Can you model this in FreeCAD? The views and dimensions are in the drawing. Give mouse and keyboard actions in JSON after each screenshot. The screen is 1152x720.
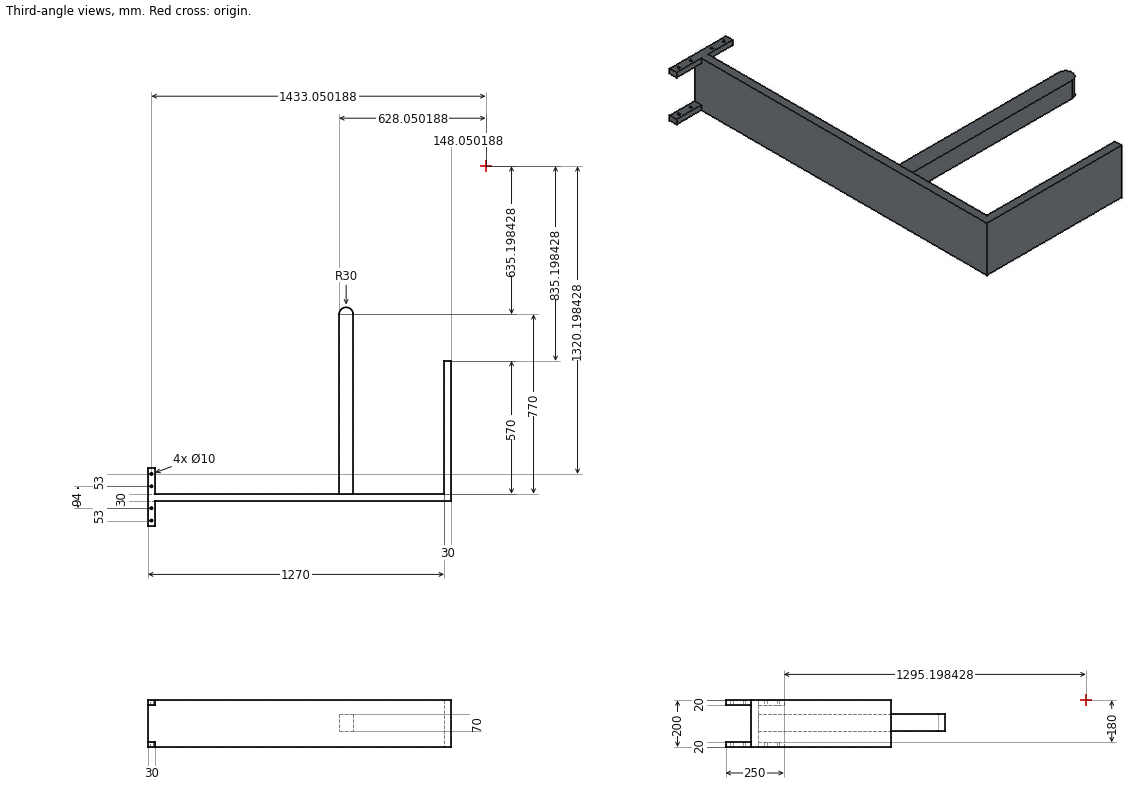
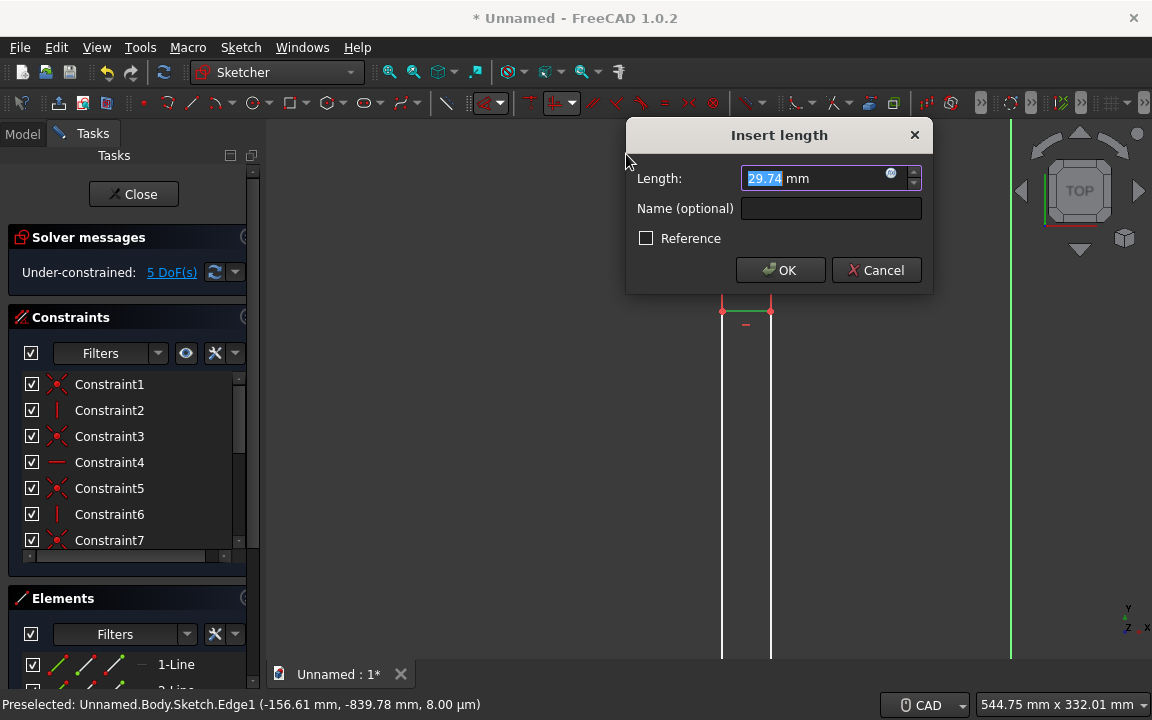
{"action": "type", "text": "30"}
{"action": "key", "text": "Return"}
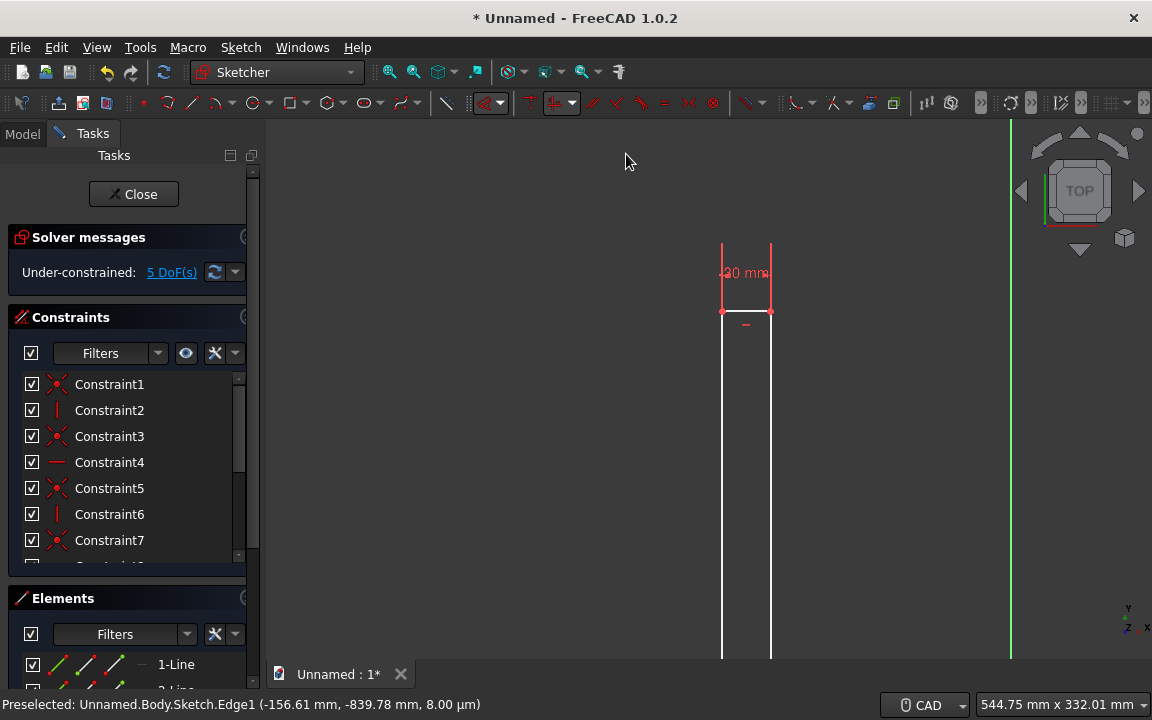
{"action": "scroll", "coordinate": [767, 432], "scroll_direction": "down", "scroll_amount": 10}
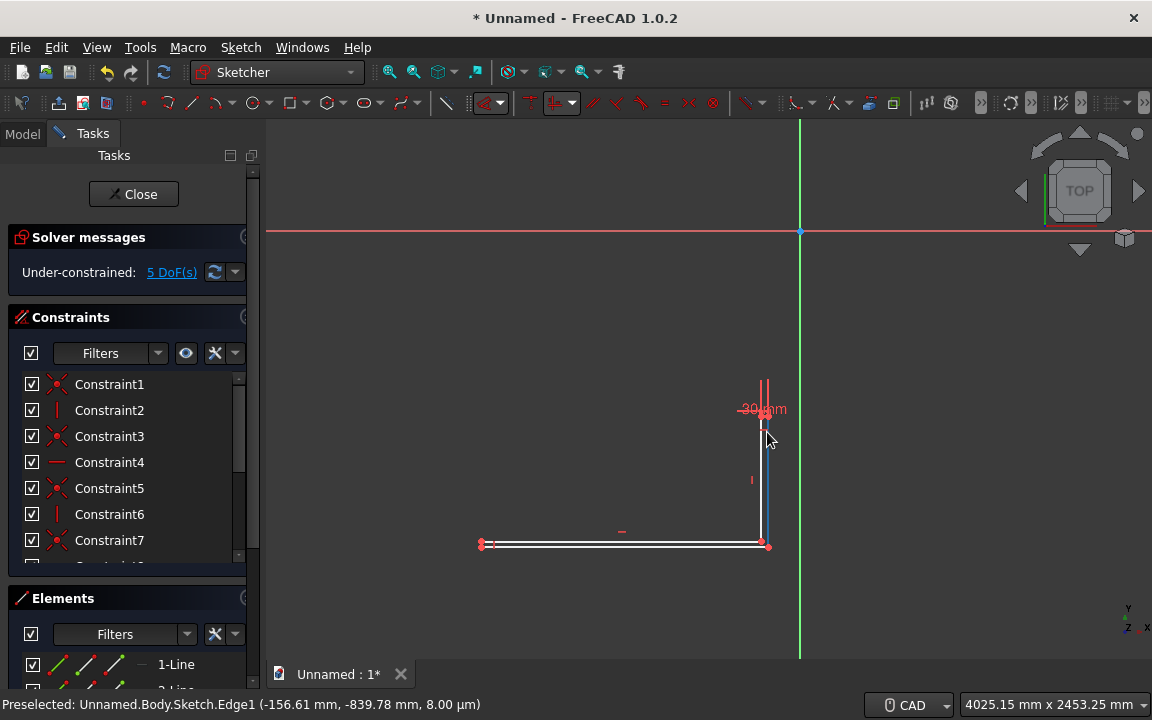
{"action": "scroll", "coordinate": [481, 544], "scroll_direction": "up", "scroll_amount": 11}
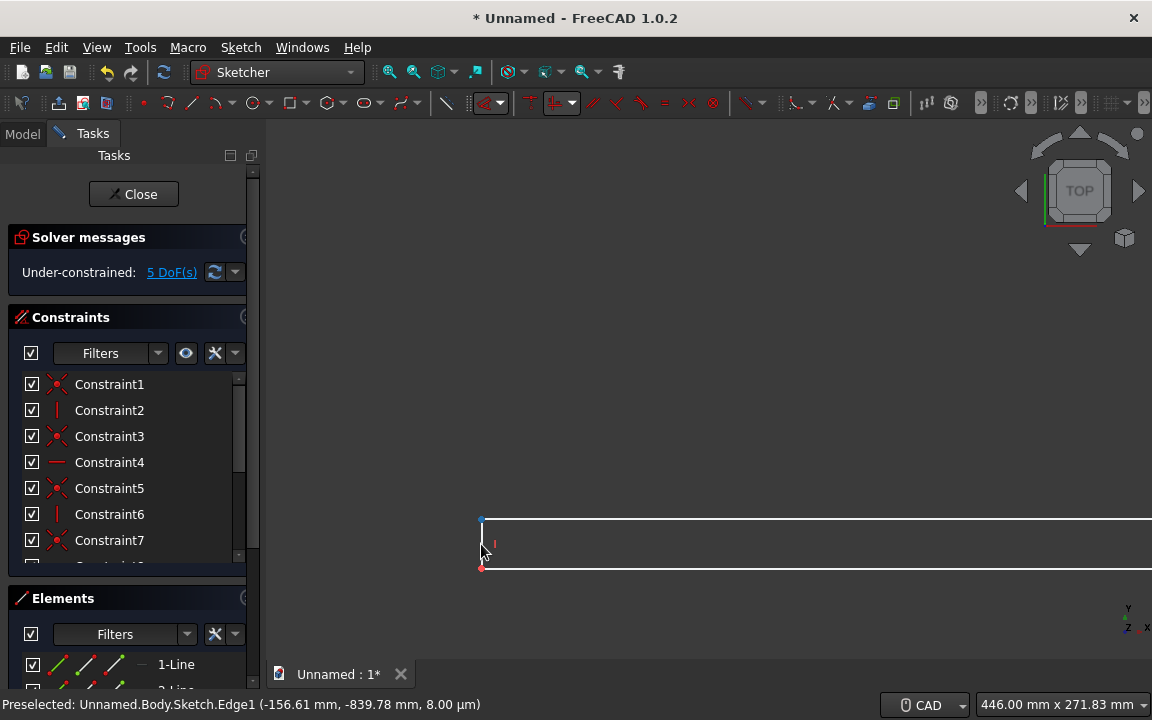
{"action": "left_click", "coordinate": [482, 534]}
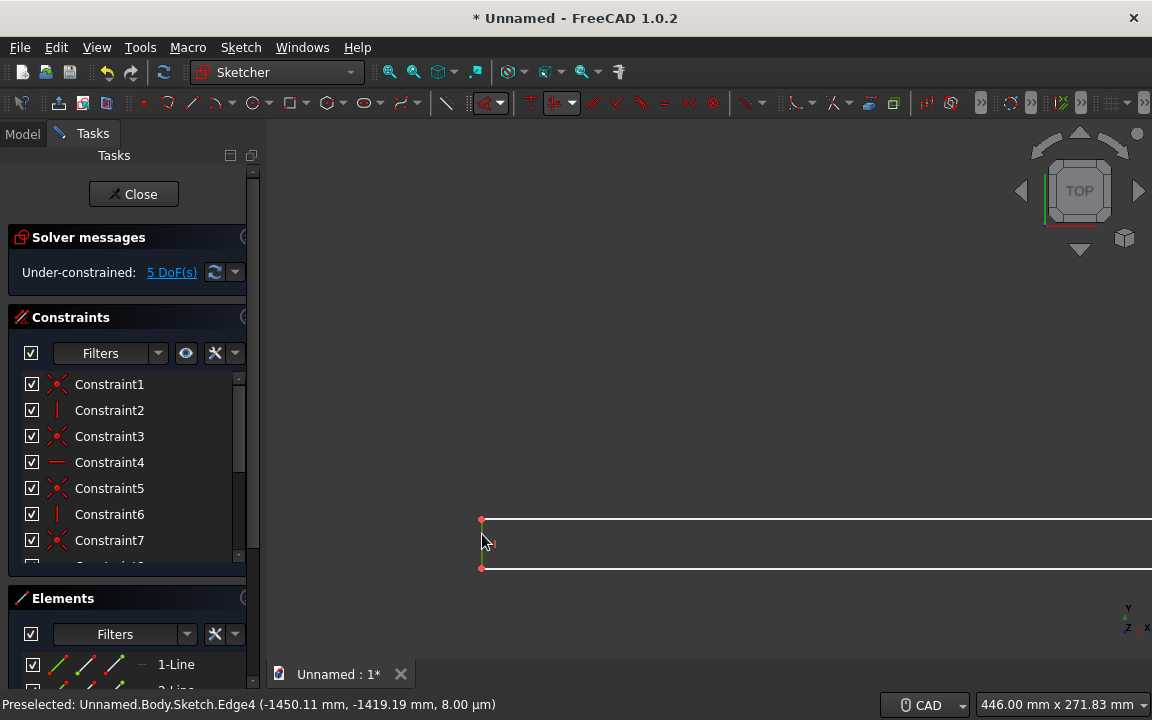
{"action": "key", "text": "i"}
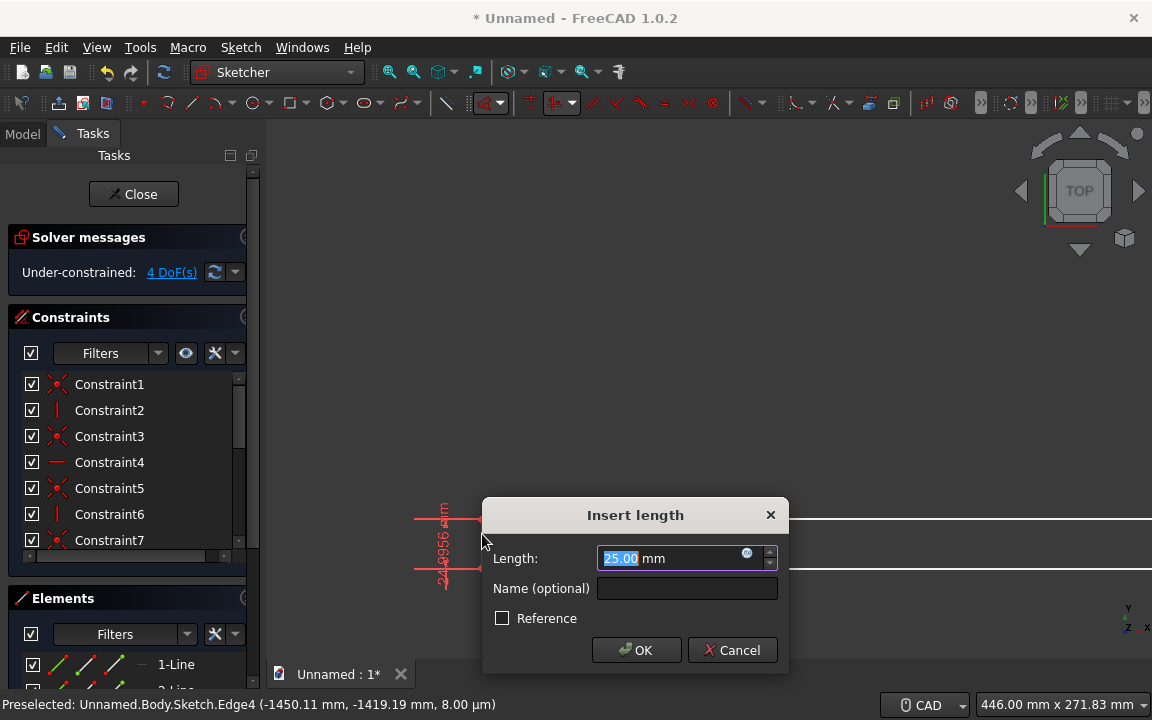
{"action": "type", "text": "30"}
{"action": "key", "text": "Return"}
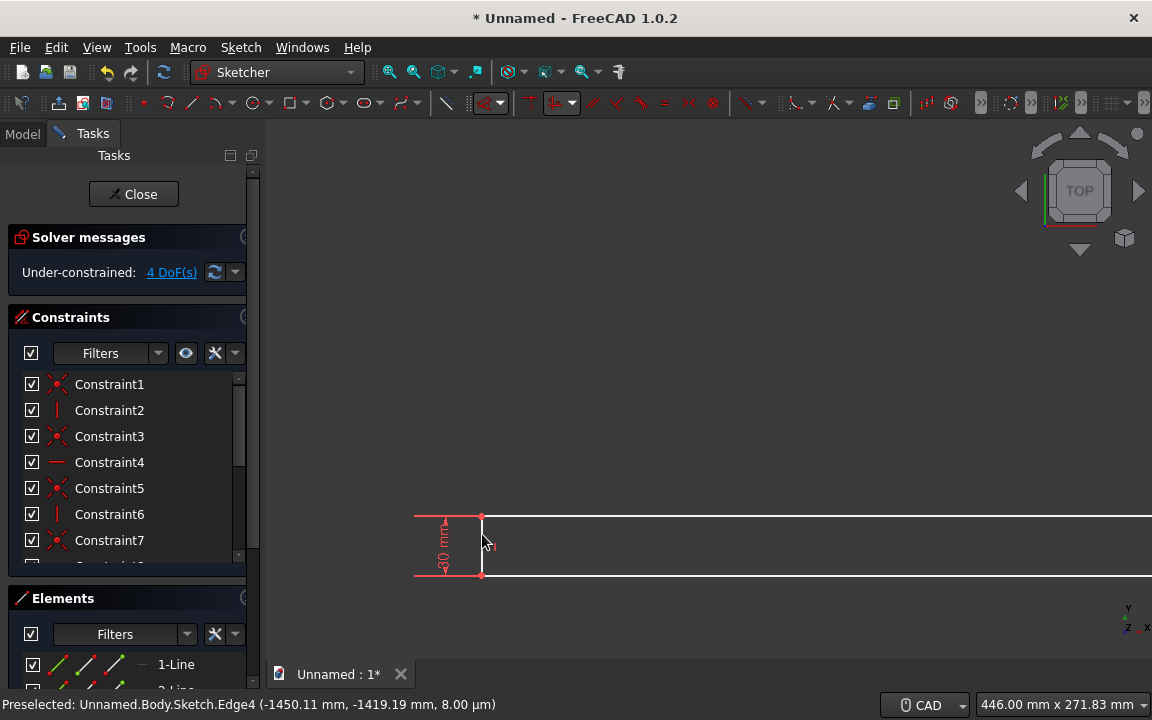
{"action": "scroll", "coordinate": [481, 544], "scroll_direction": "down", "scroll_amount": 11}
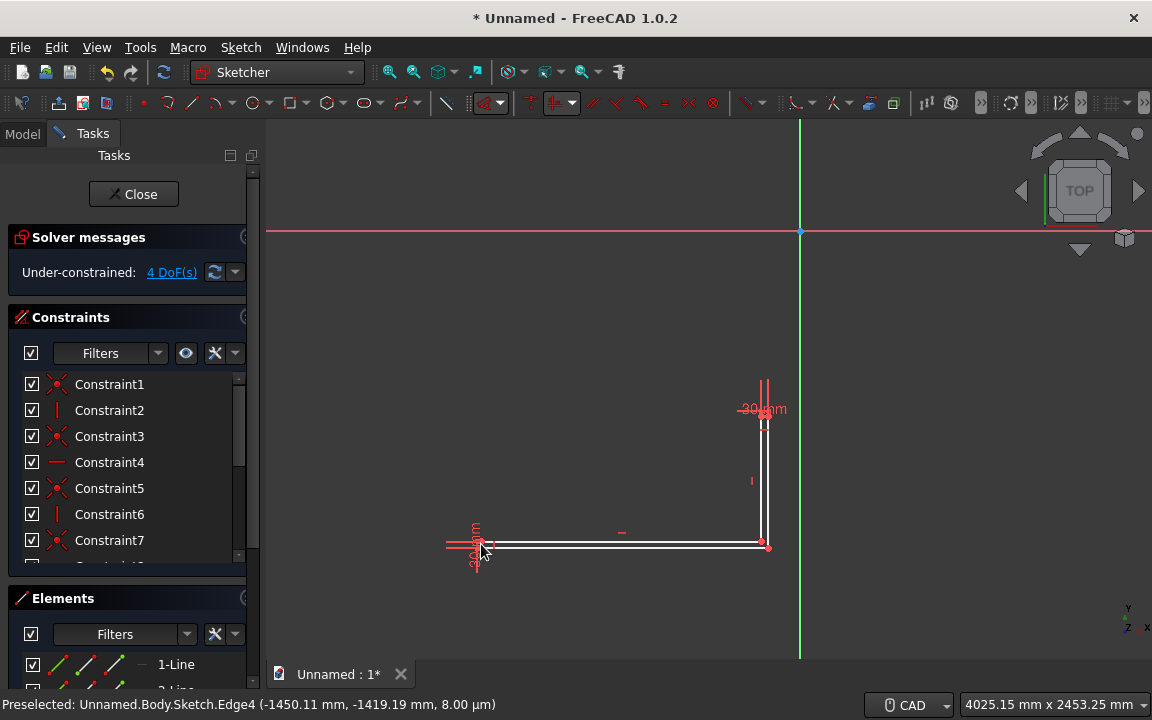
{"action": "scroll", "coordinate": [761, 454], "scroll_direction": "up", "scroll_amount": 4}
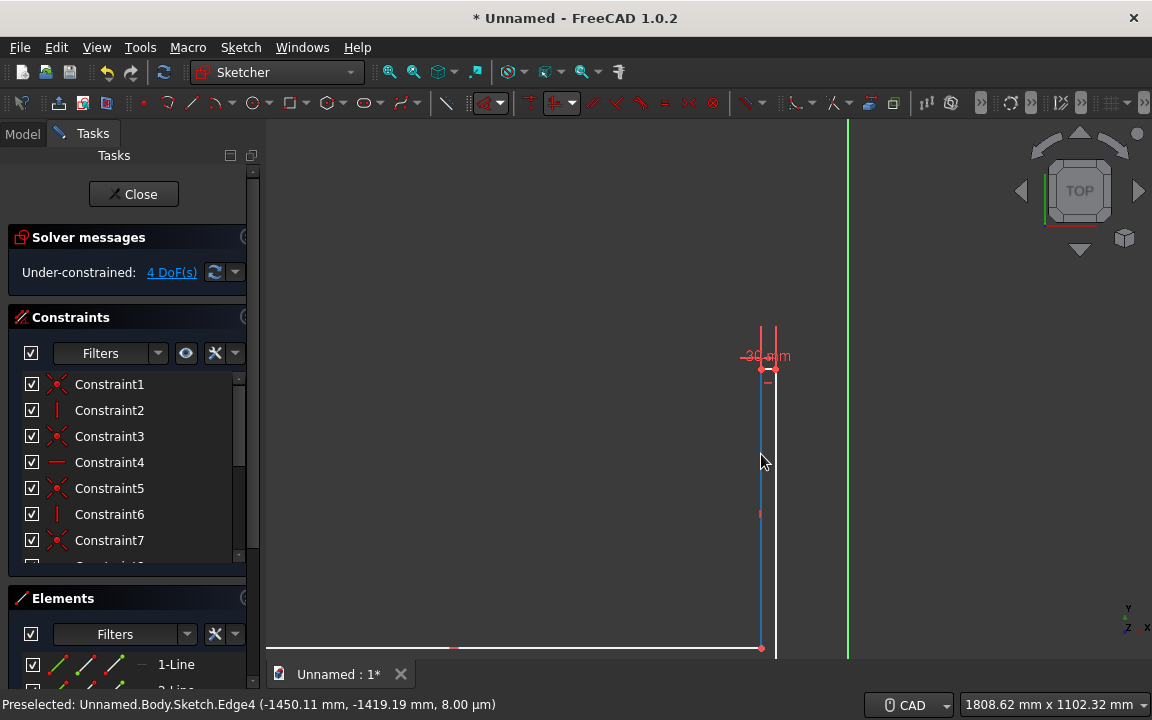
{"action": "left_click", "coordinate": [761, 453]}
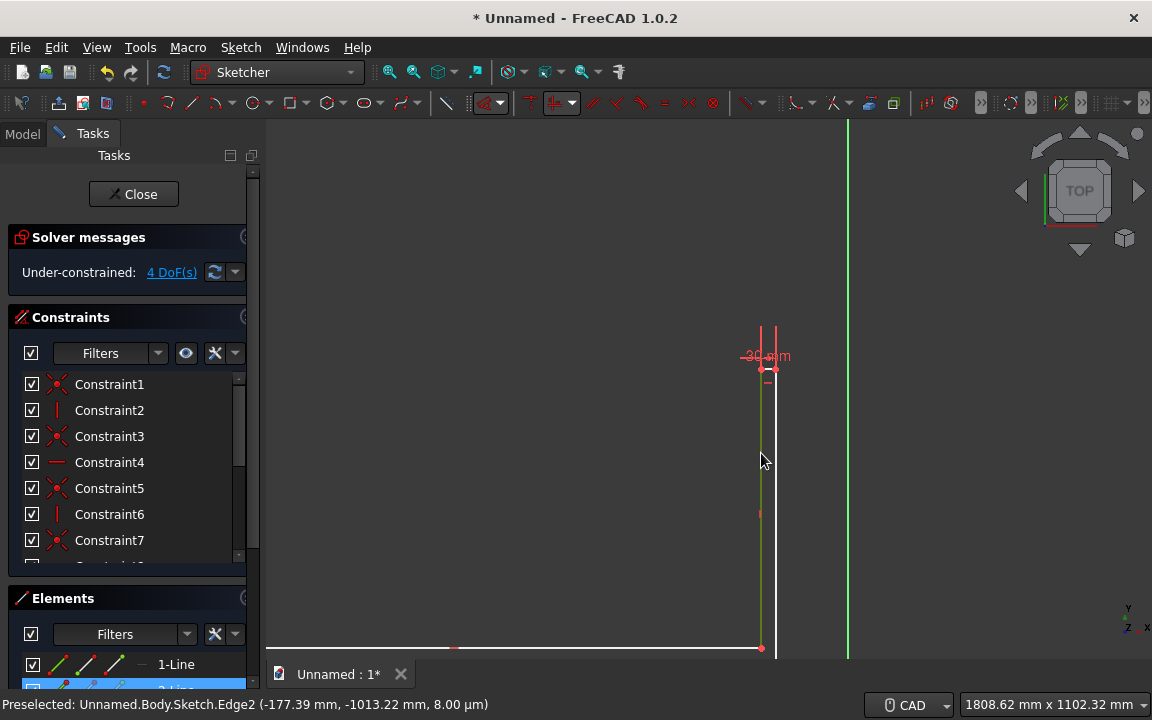
{"action": "key", "text": "i"}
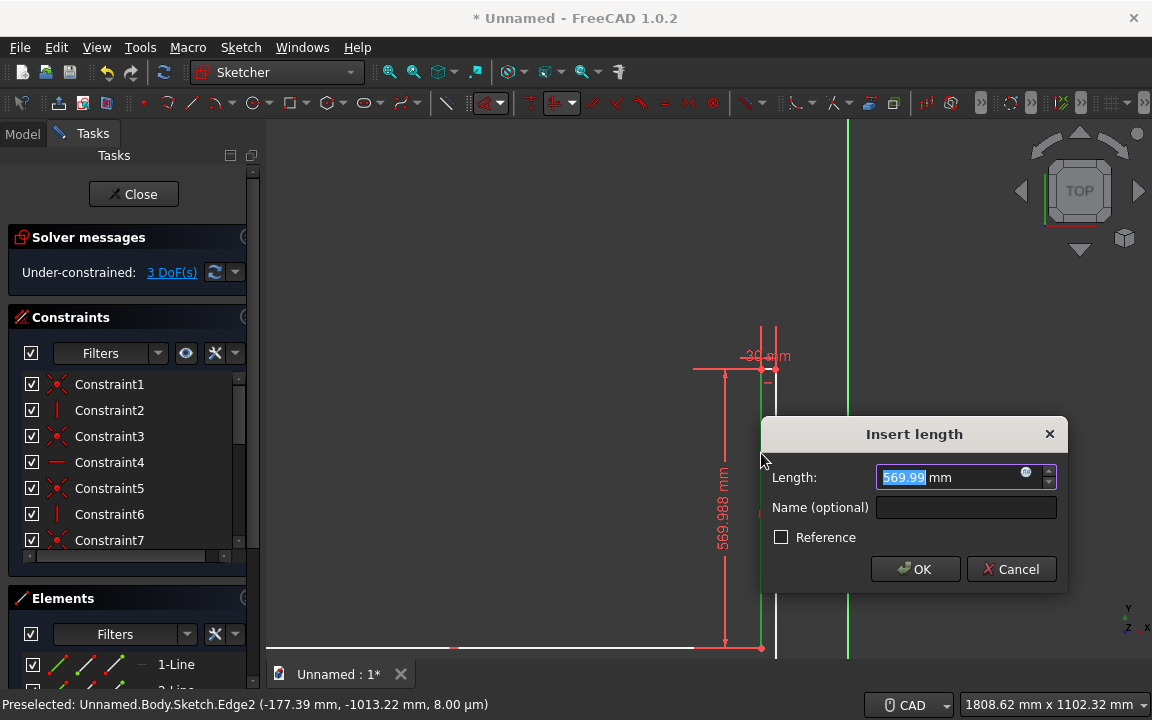
{"action": "type", "text": "570"}
{"action": "key", "text": "Return"}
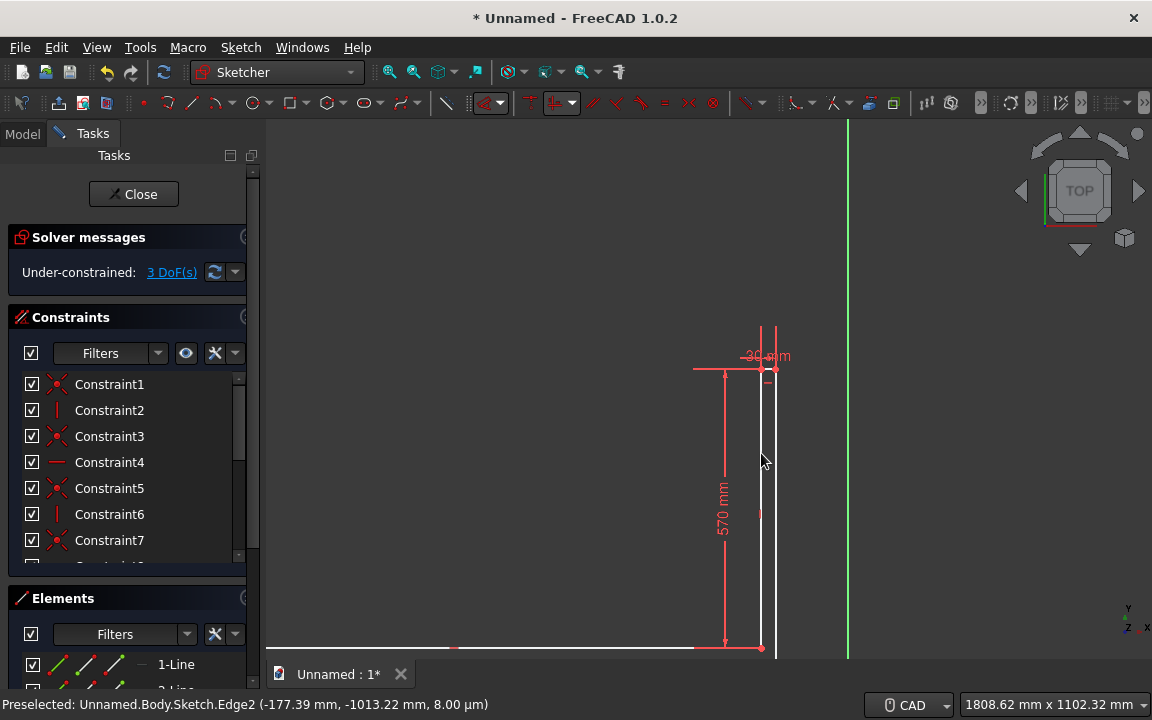
{"action": "scroll", "coordinate": [760, 454], "scroll_direction": "down", "scroll_amount": 4}